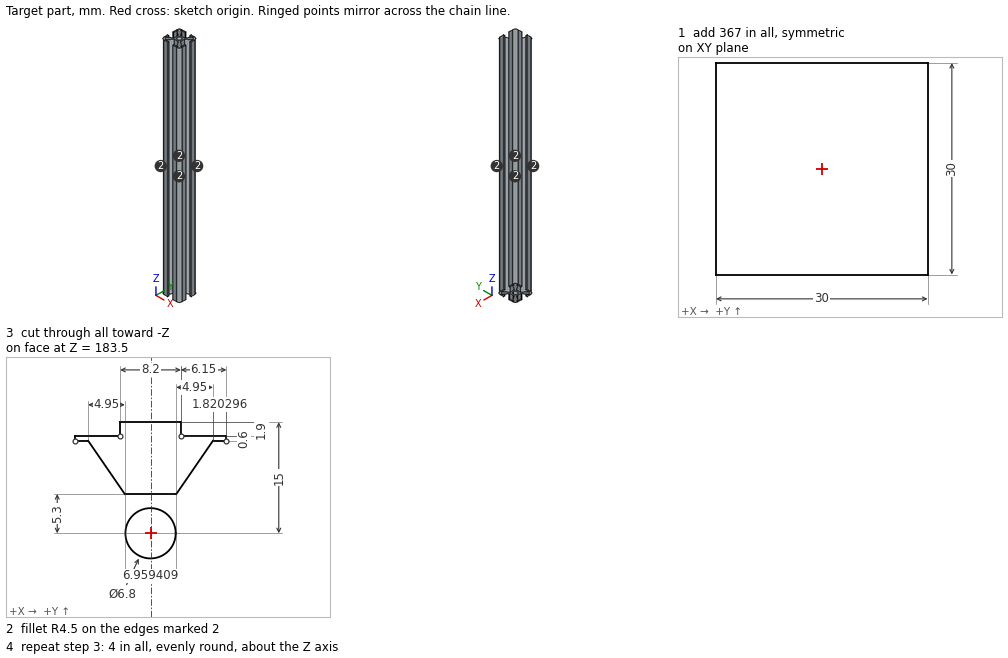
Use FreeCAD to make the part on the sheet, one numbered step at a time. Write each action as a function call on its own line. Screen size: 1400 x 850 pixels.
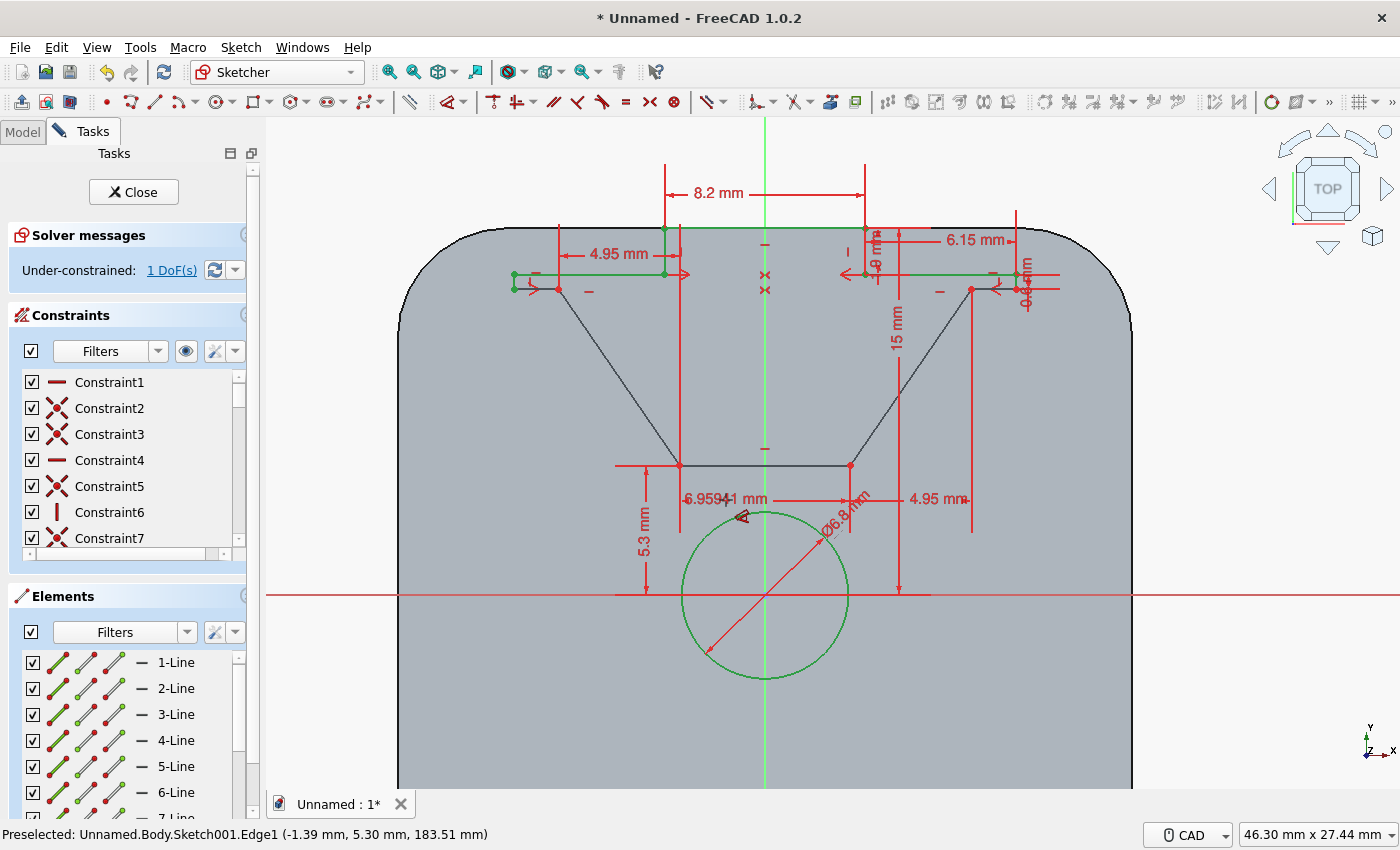
click(985, 289)
click(994, 323)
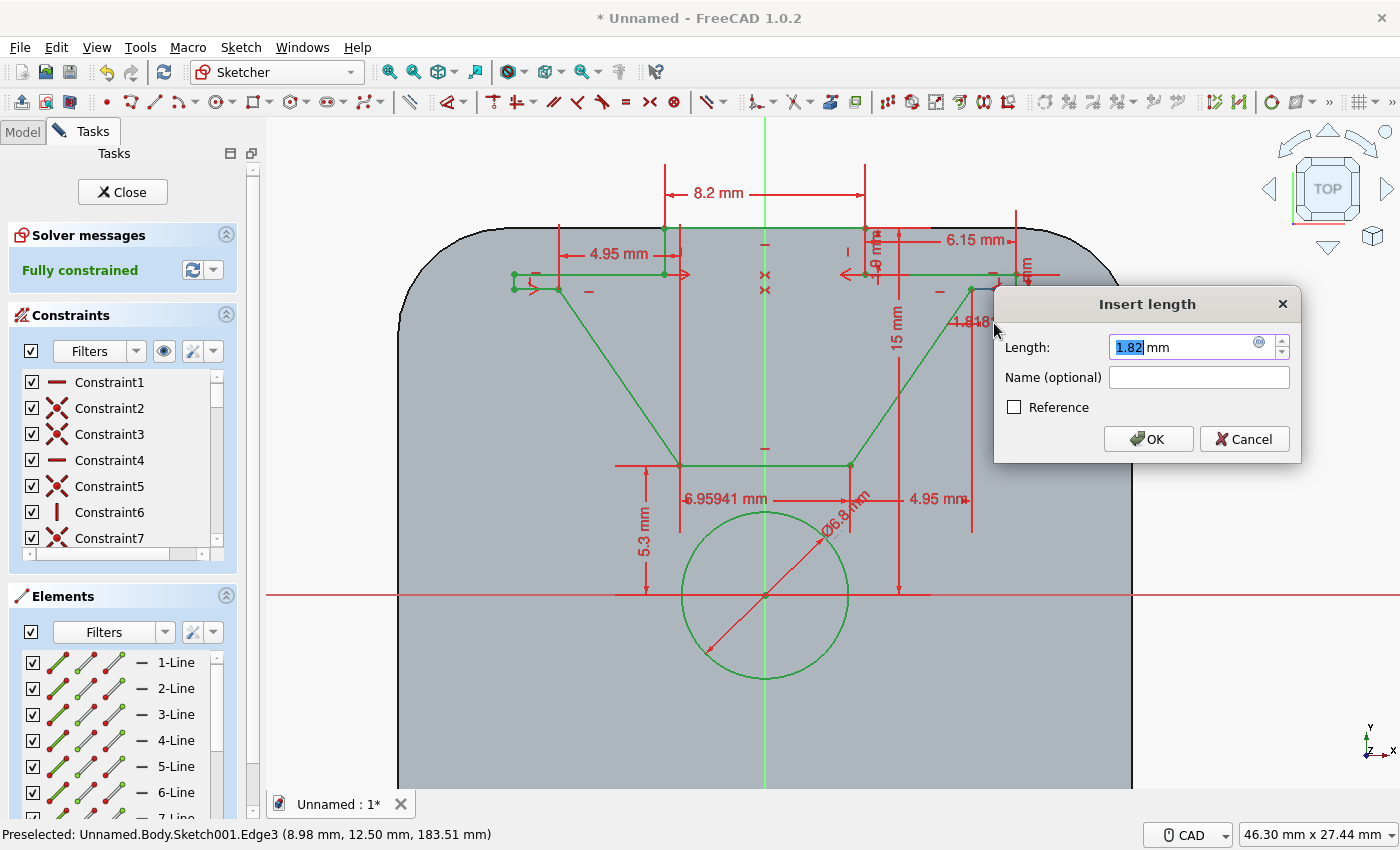
text(1.820296)
key(Return)
key(Escape)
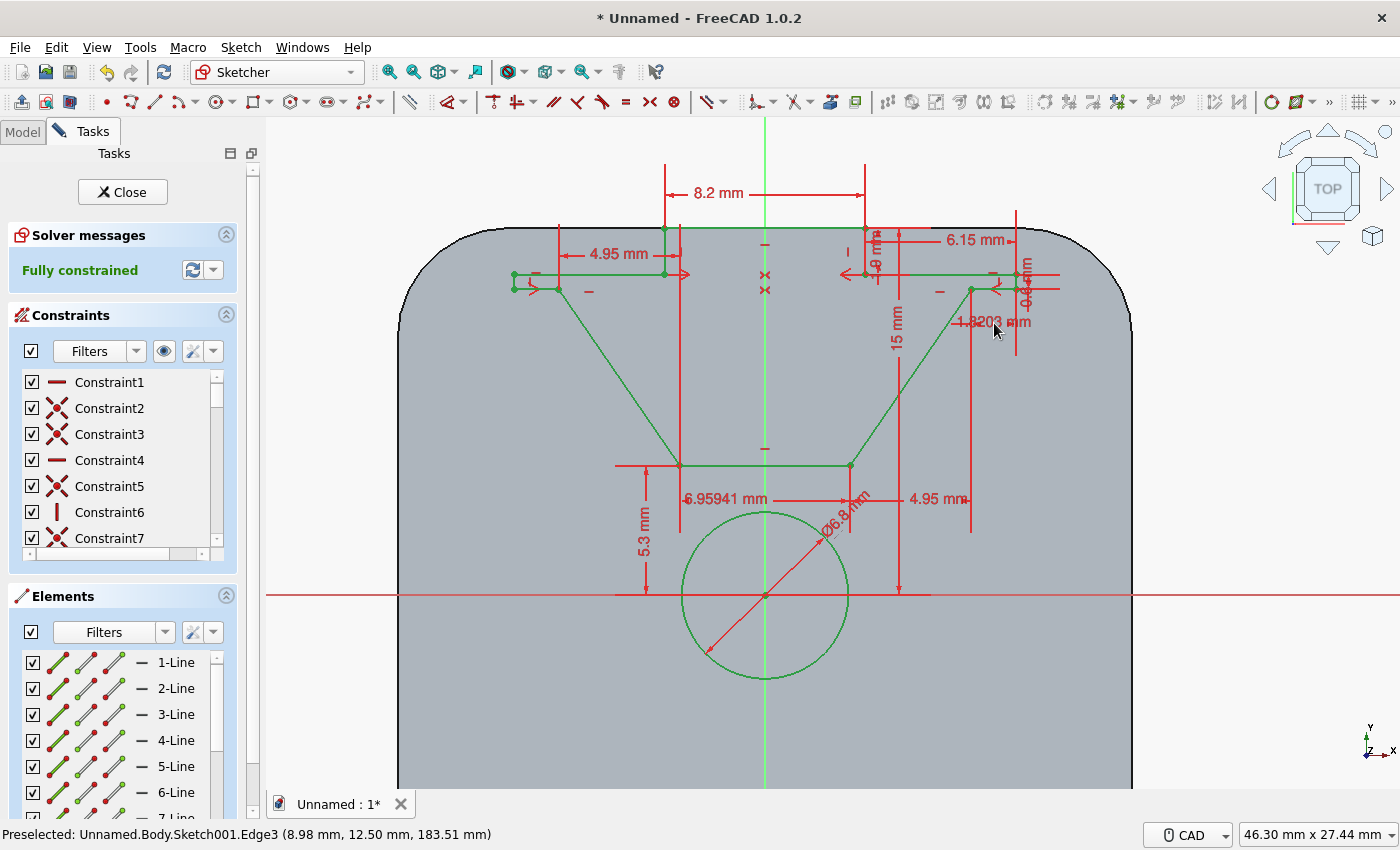
click(123, 192)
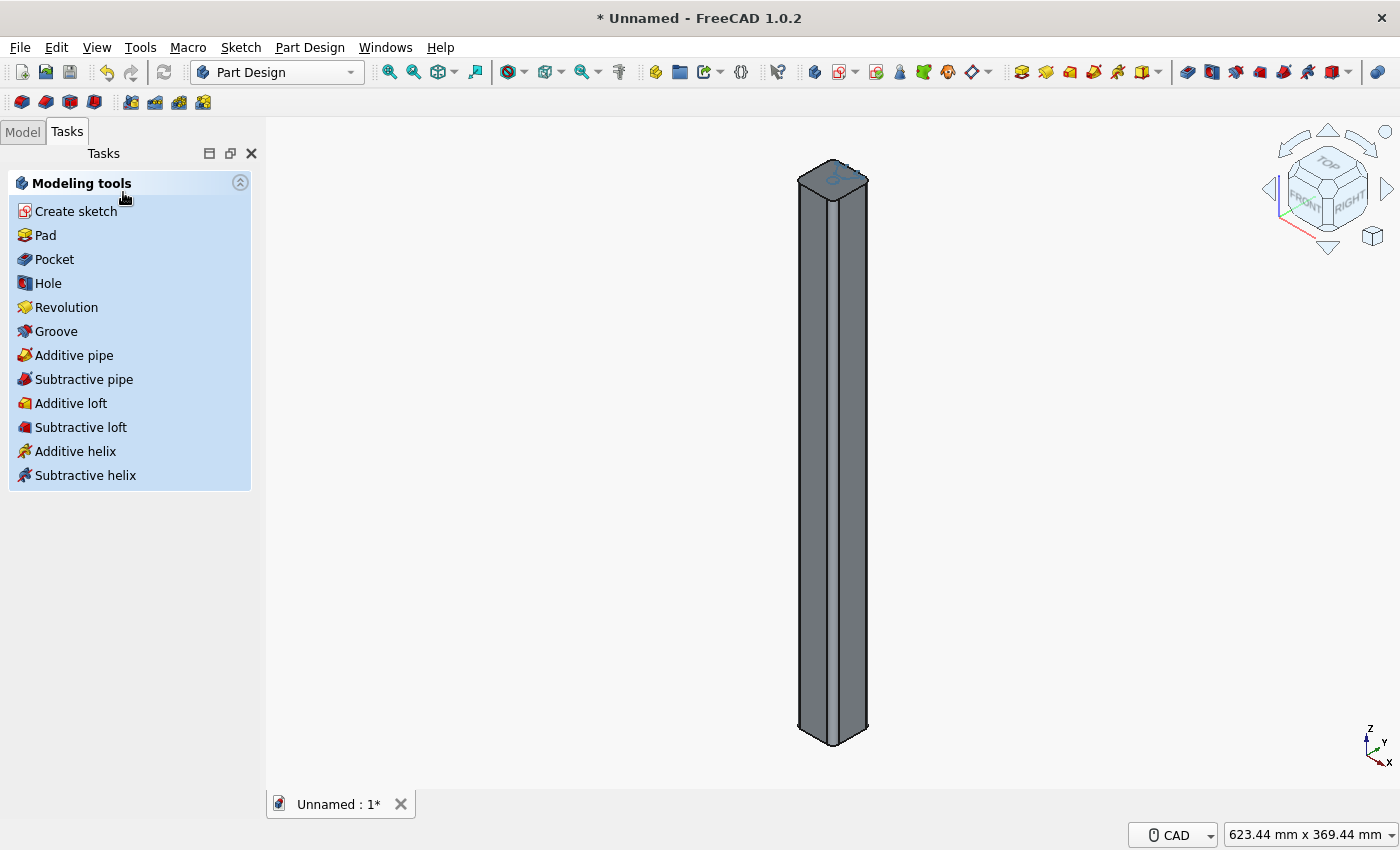
click(1188, 72)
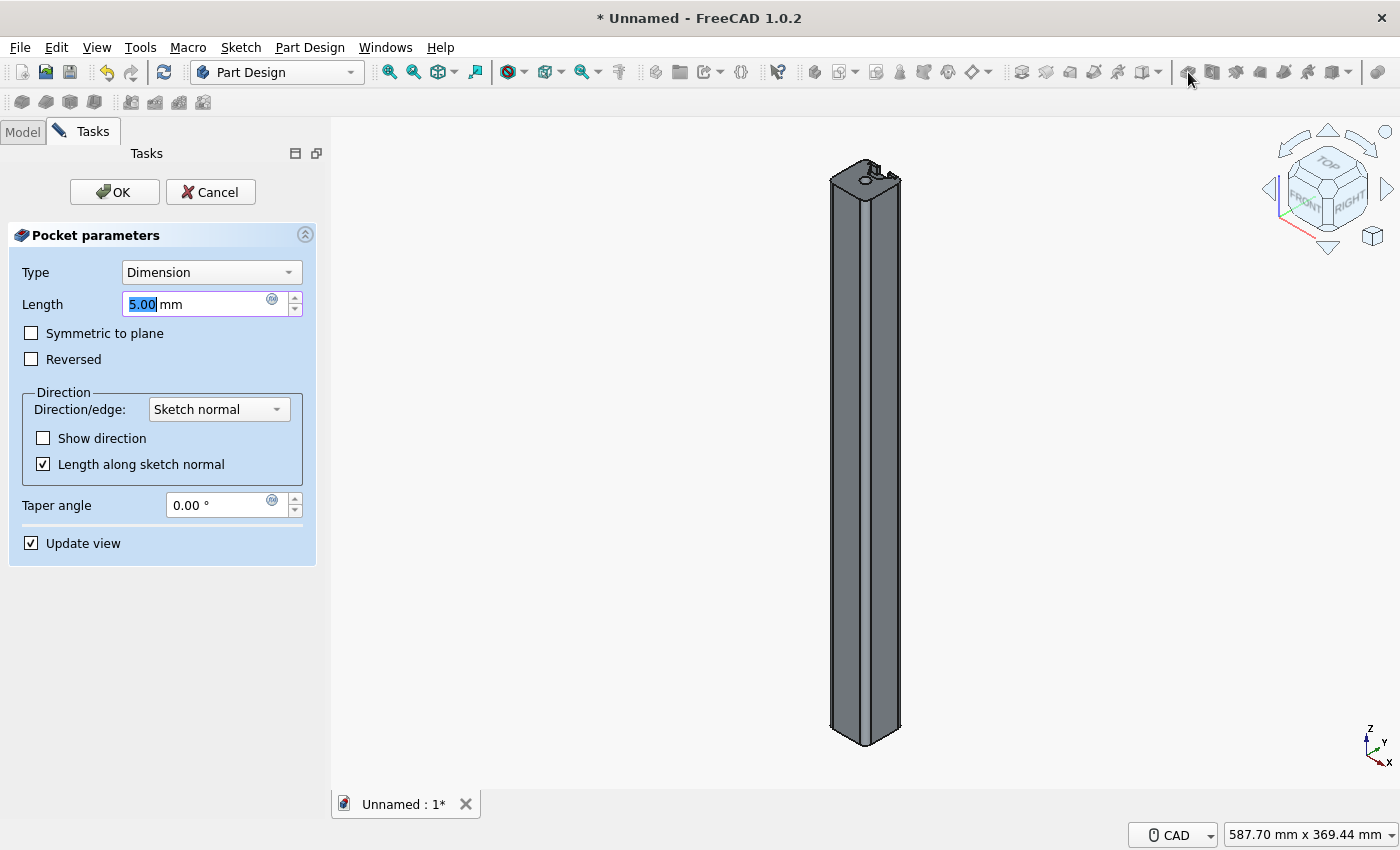
click(212, 272)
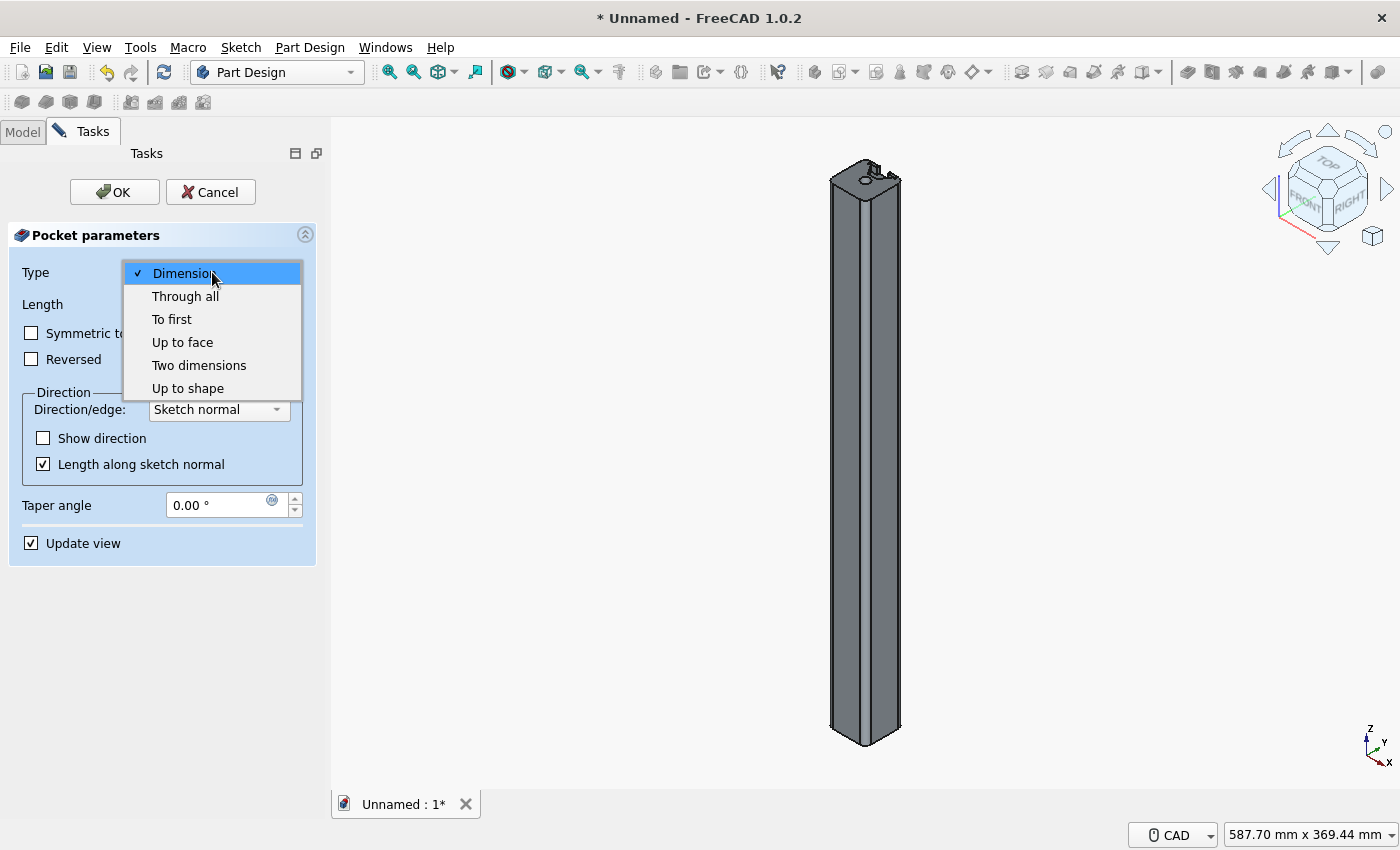
click(212, 296)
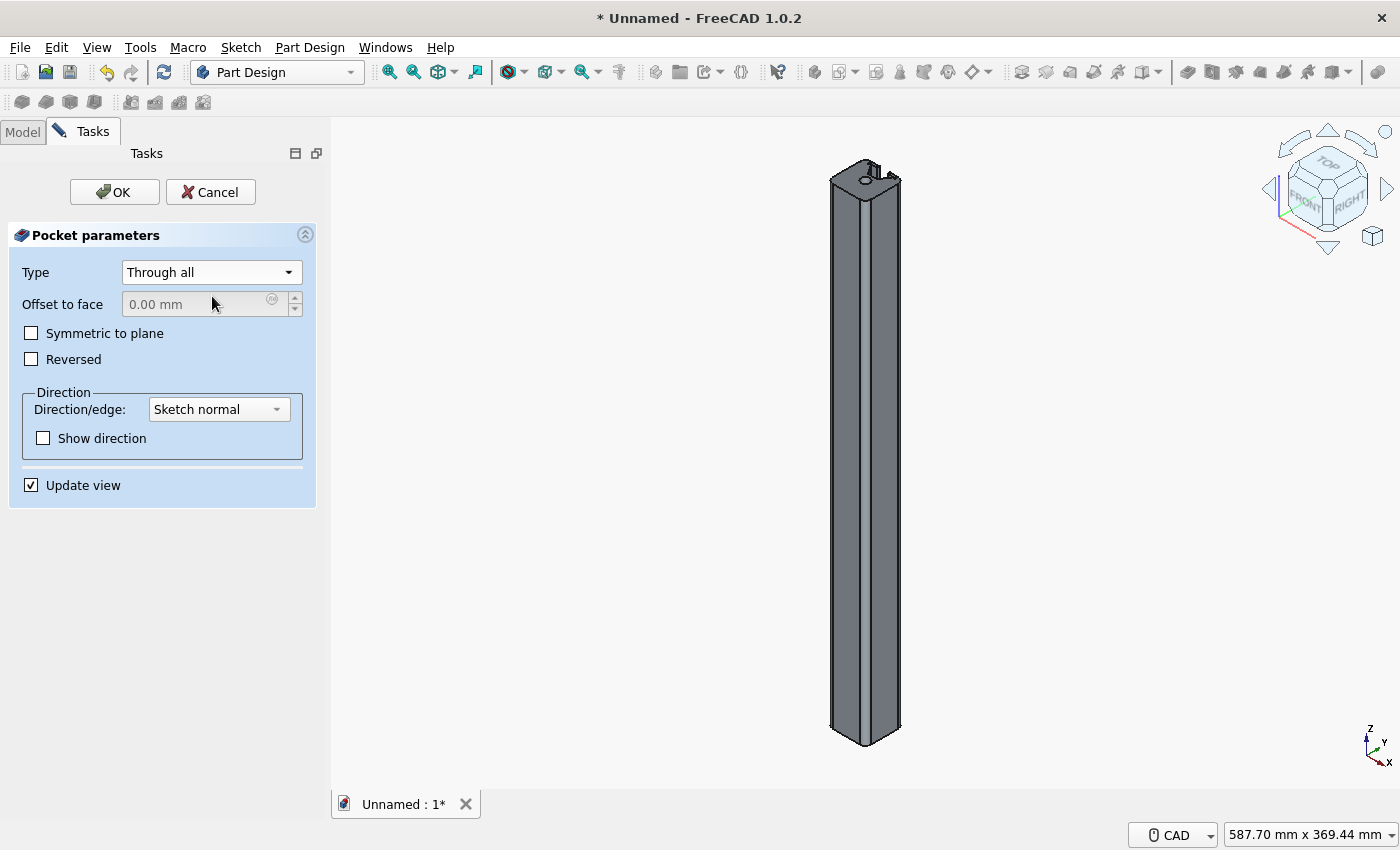
click(115, 192)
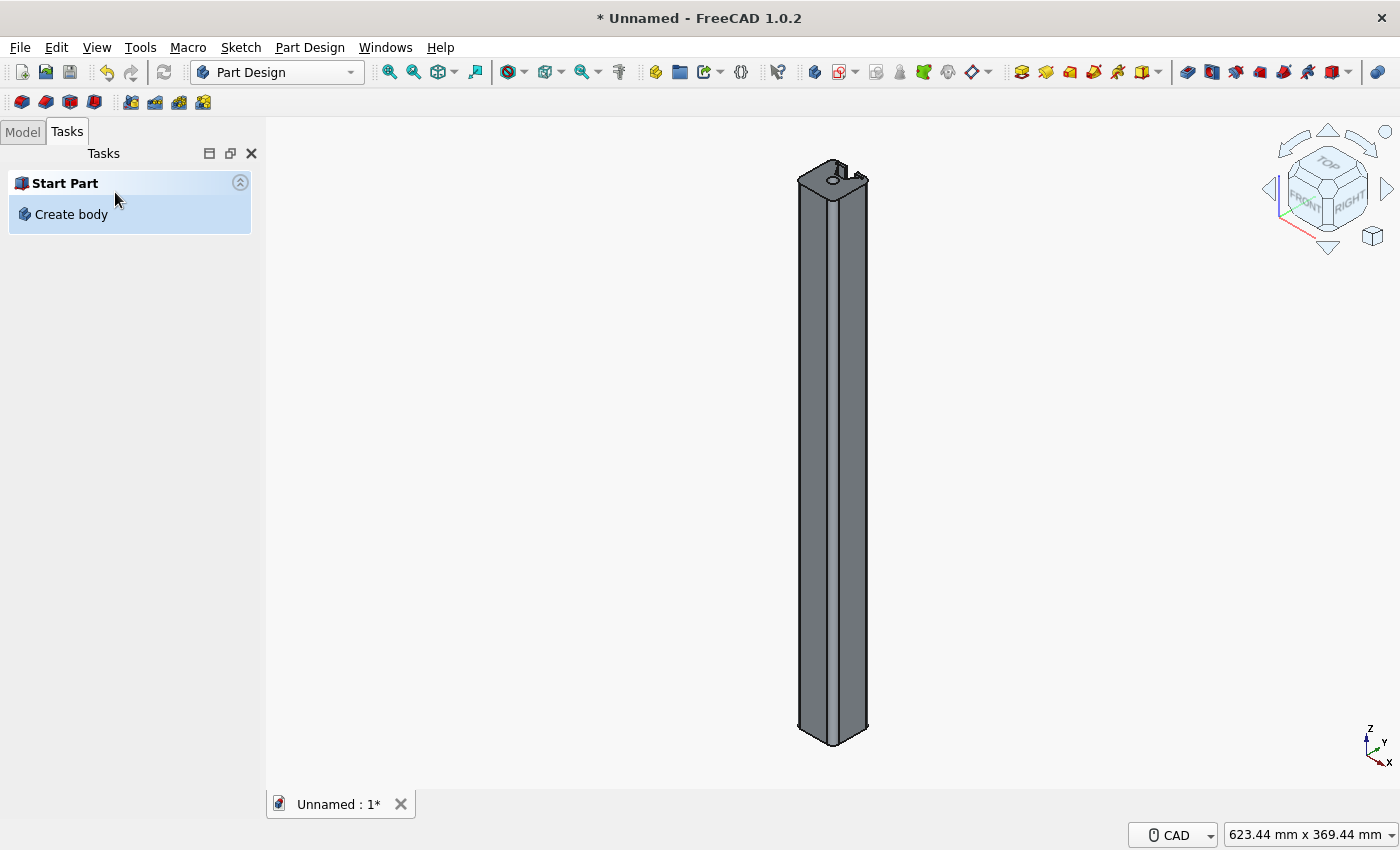
click(23, 131)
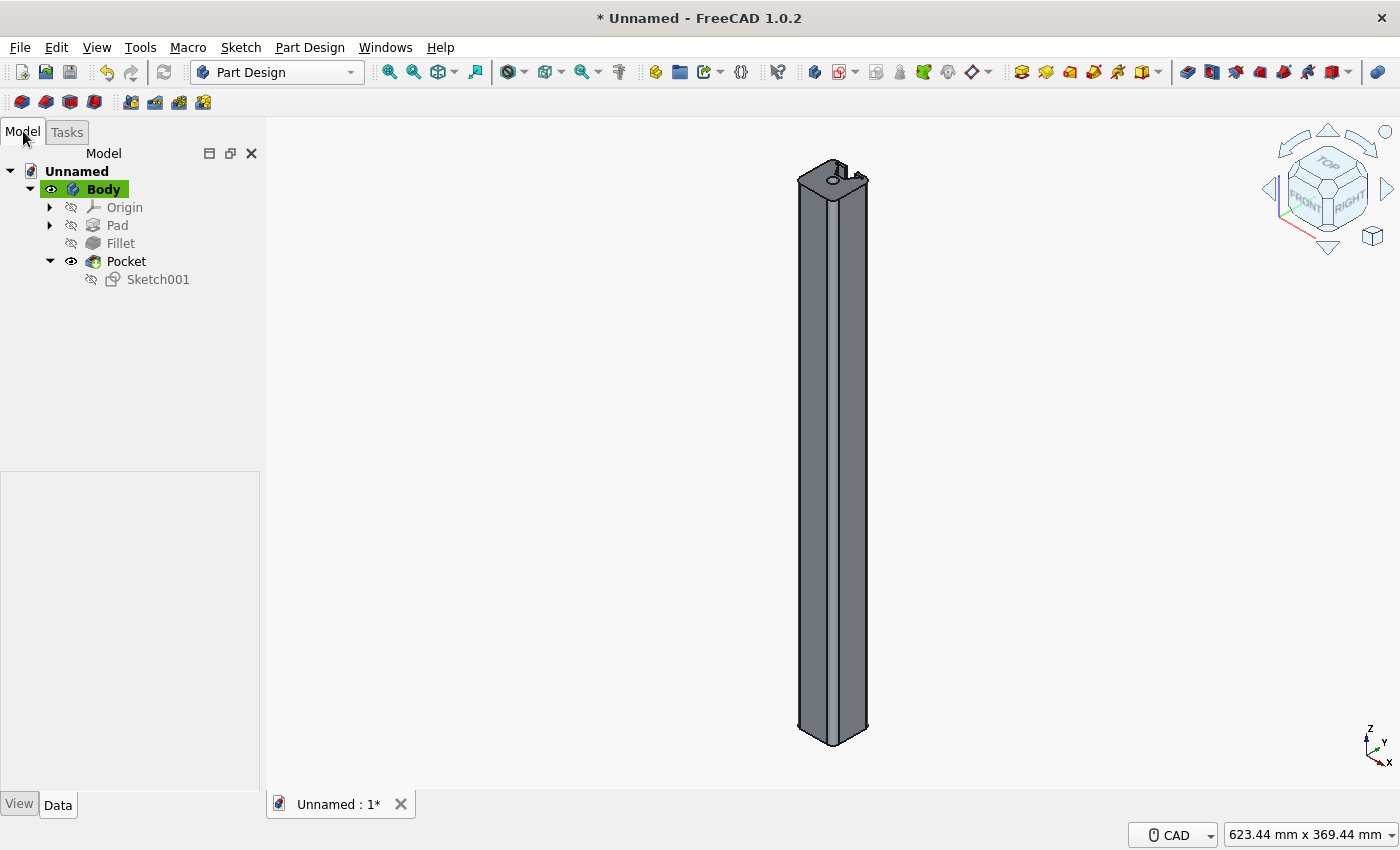
click(116, 261)